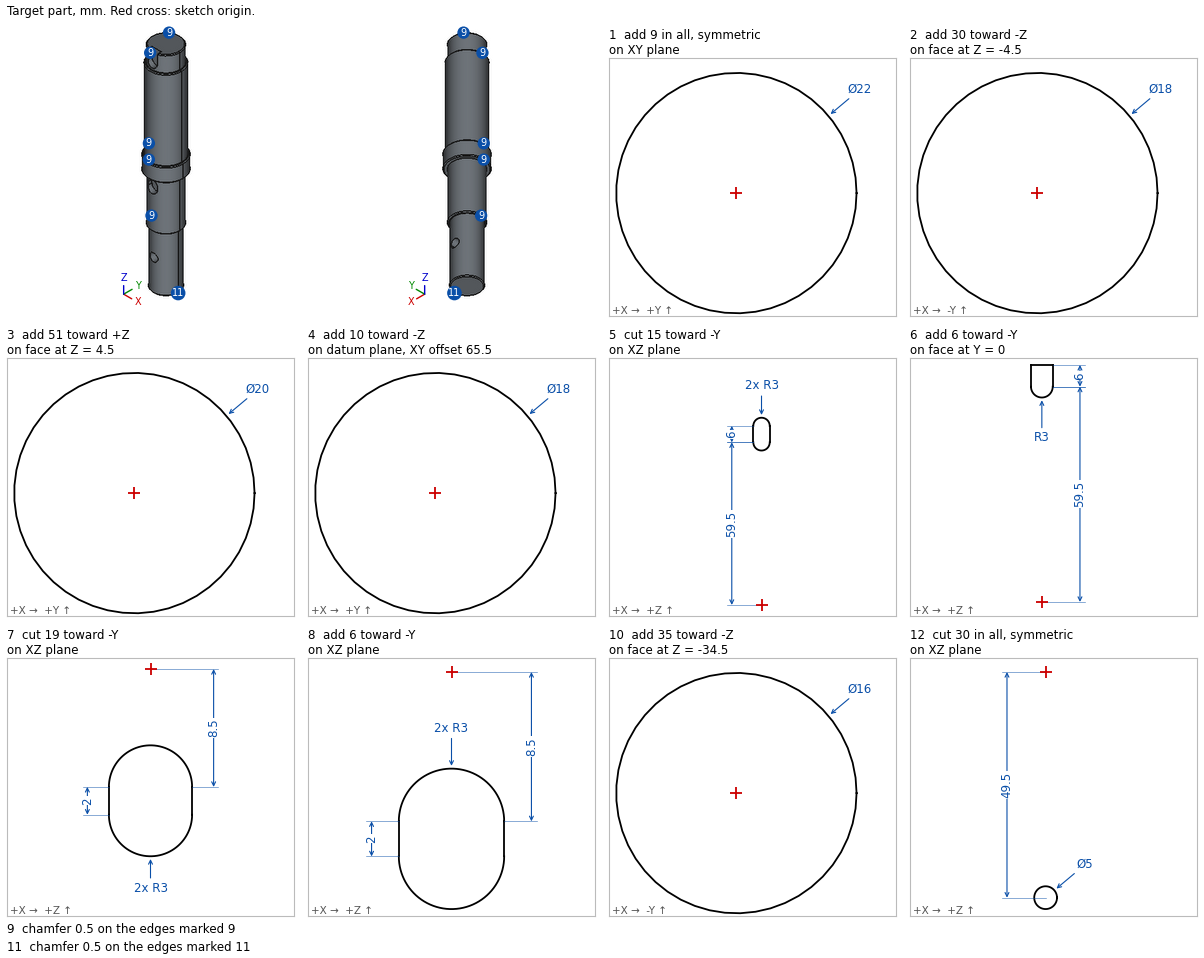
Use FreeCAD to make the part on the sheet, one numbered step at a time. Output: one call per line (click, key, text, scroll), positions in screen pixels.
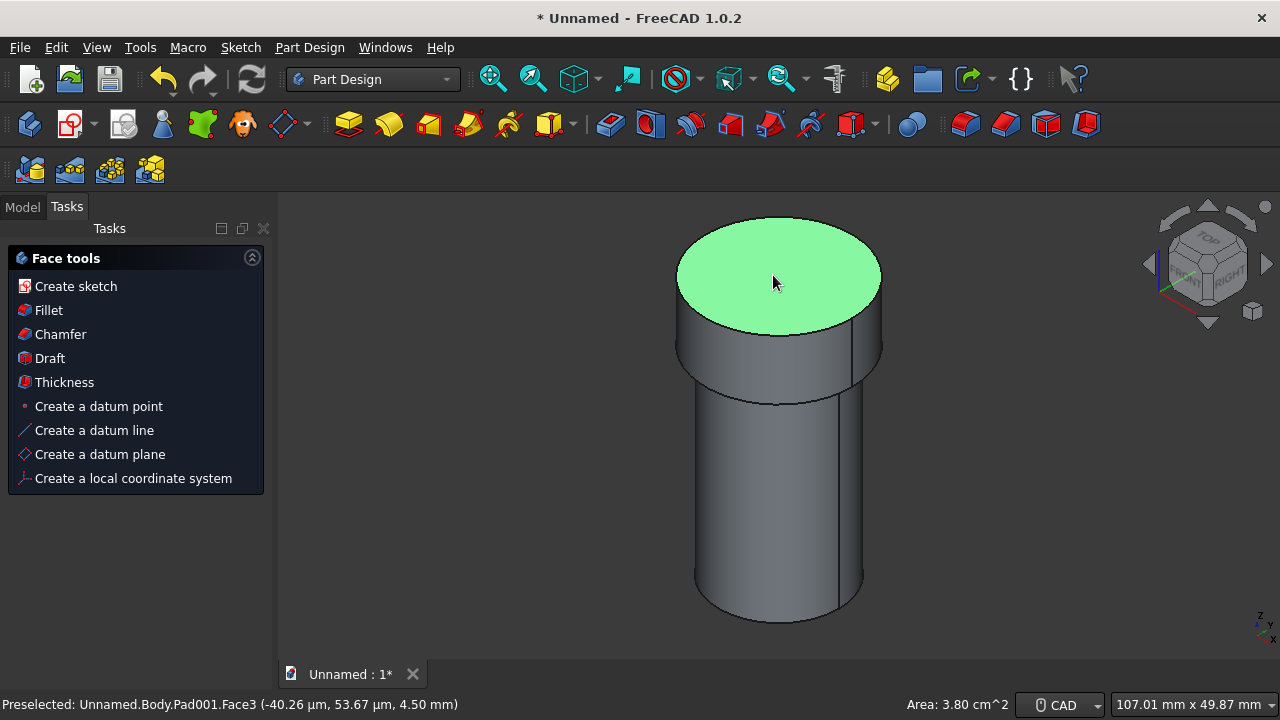
click(70, 124)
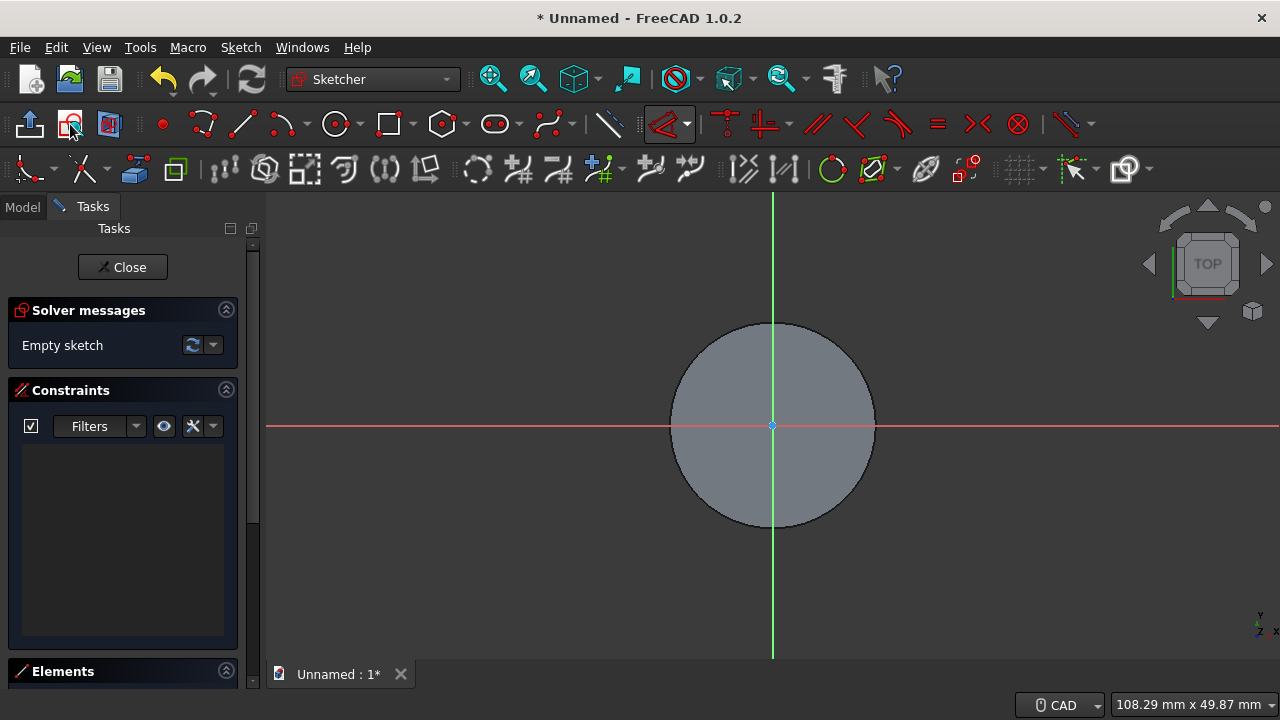
scroll(912, 425, up, 2)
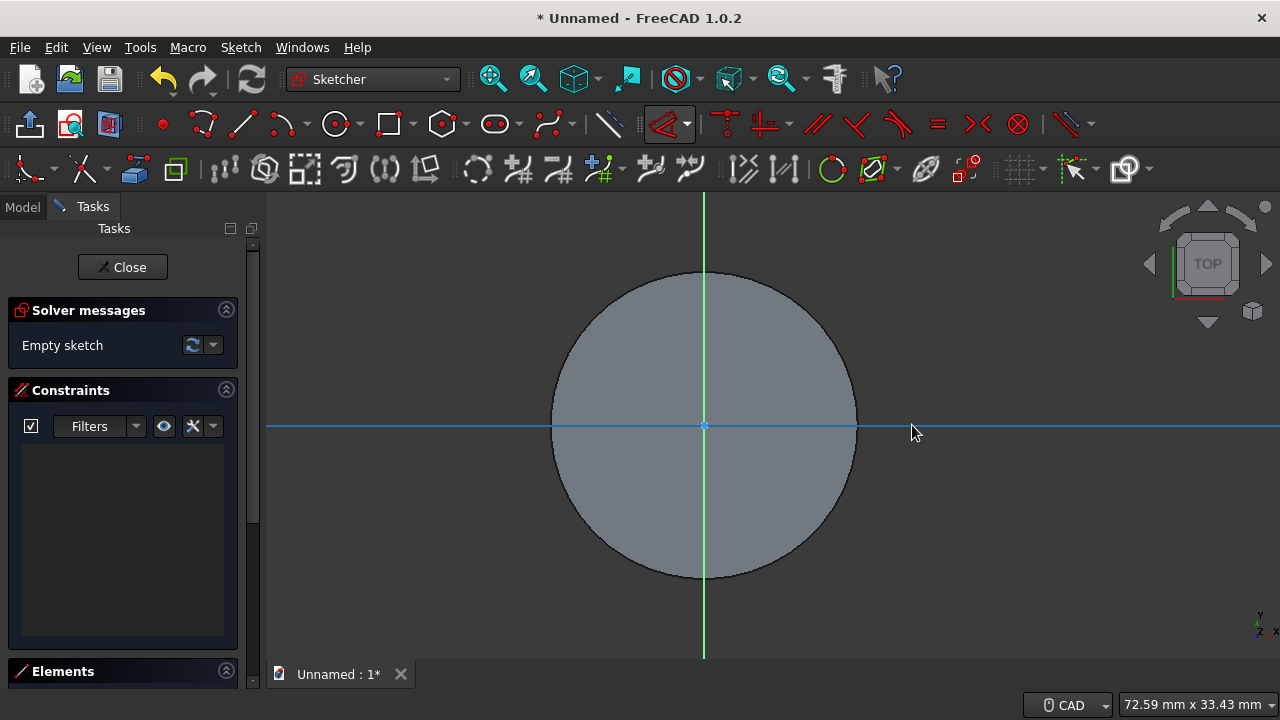
click(336, 124)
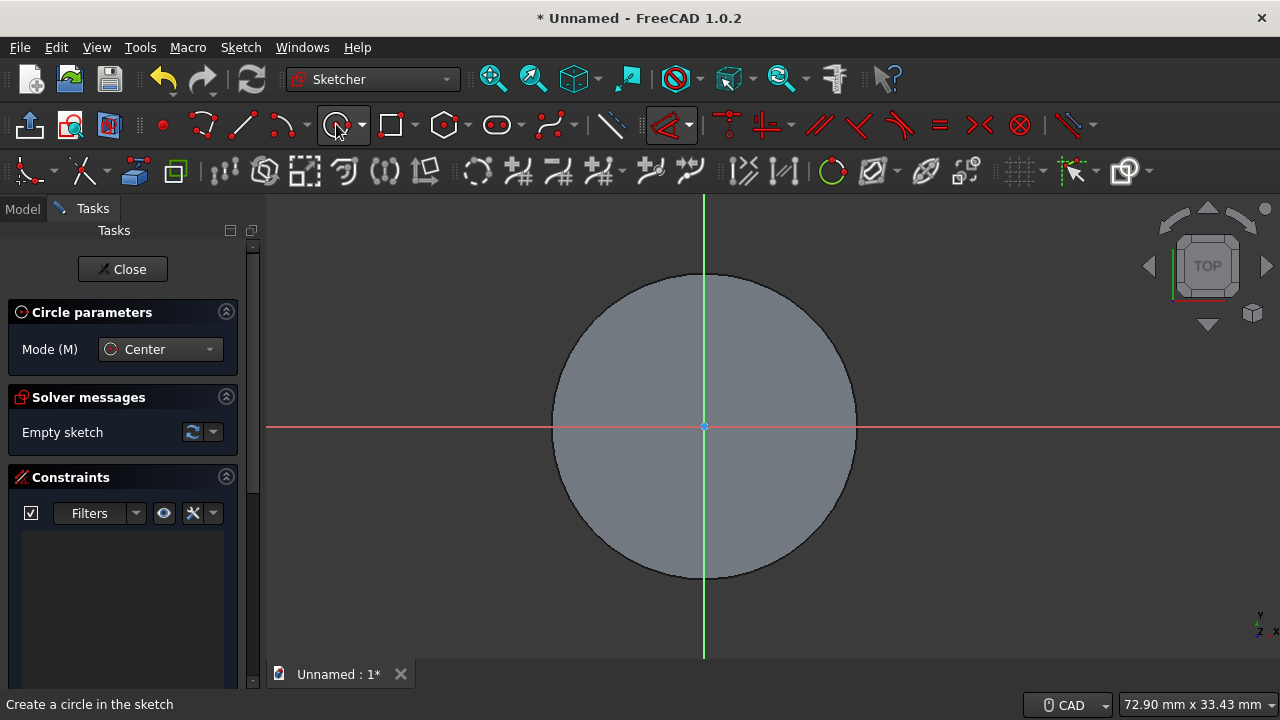
click(704, 426)
click(803, 328)
key(Escape)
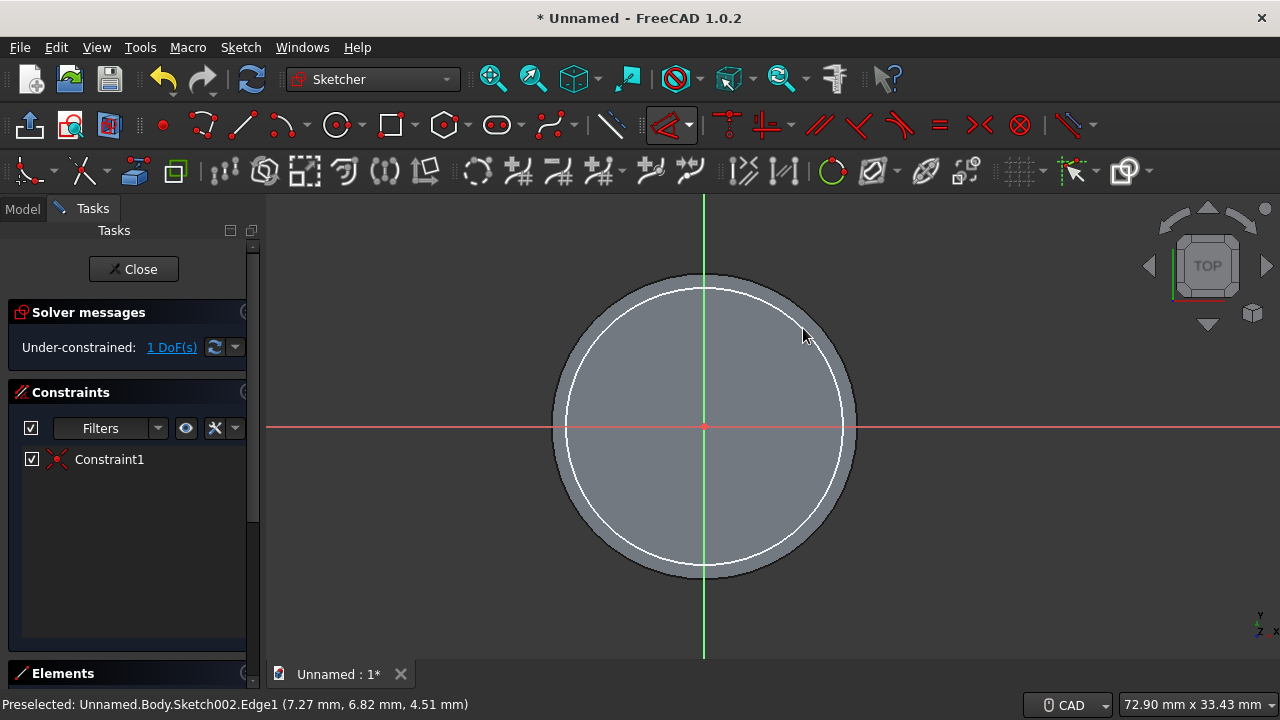
click(802, 328)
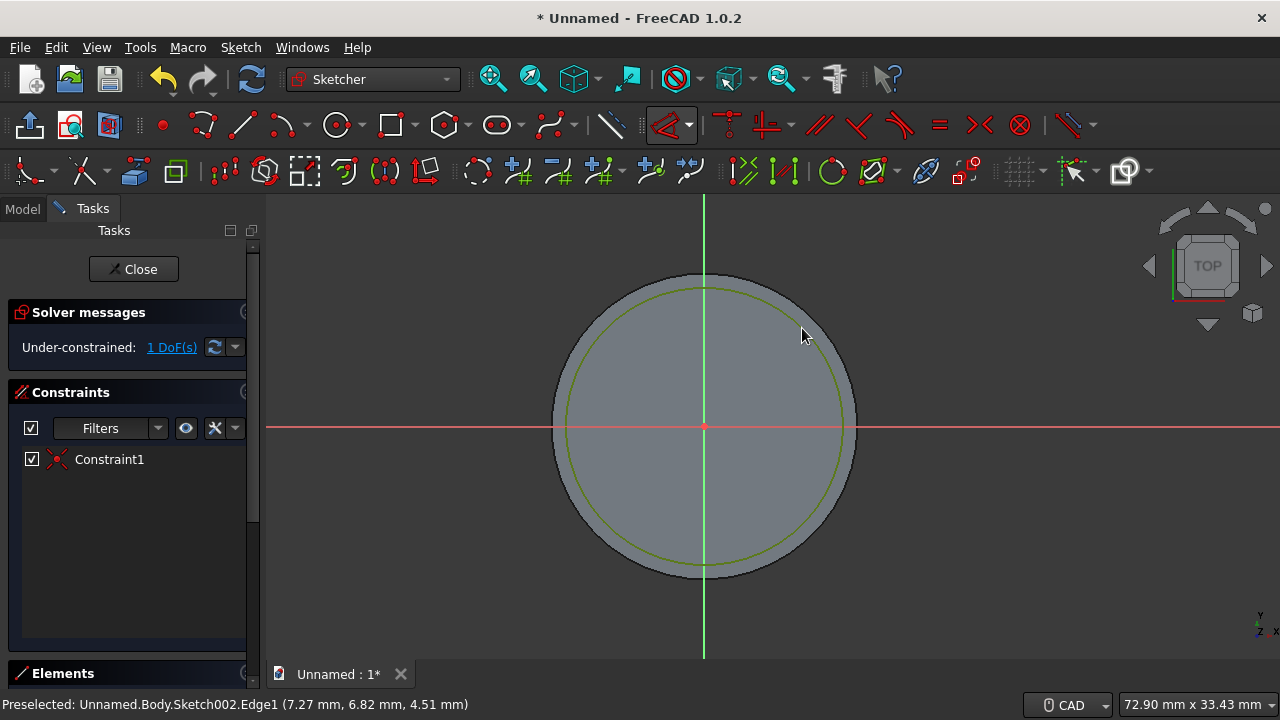
key(k)
key(o)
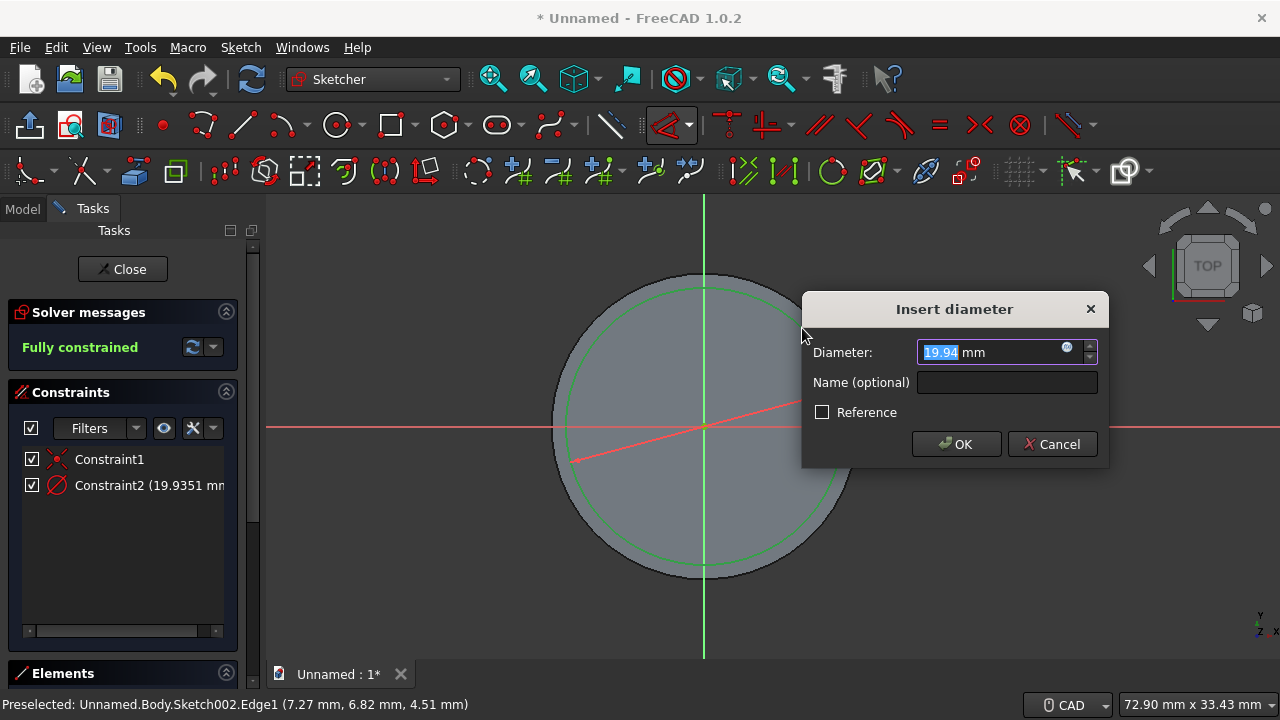
text(20)
key(Return)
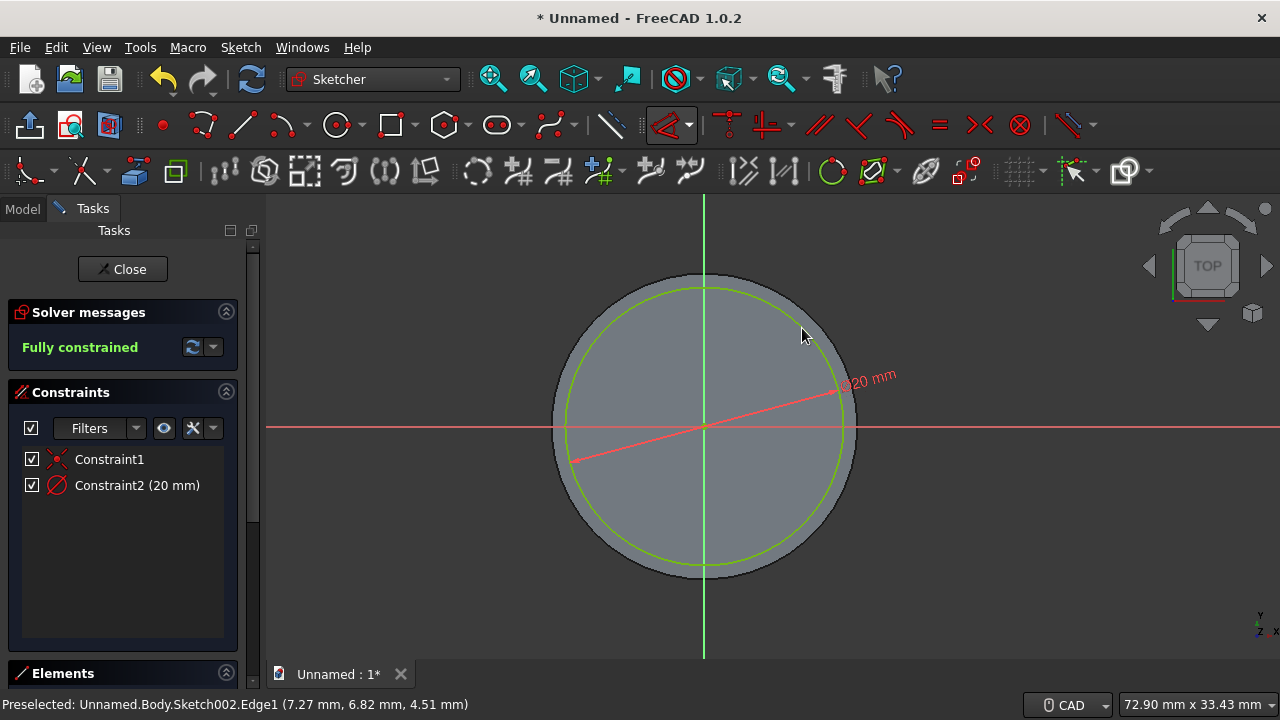
click(123, 269)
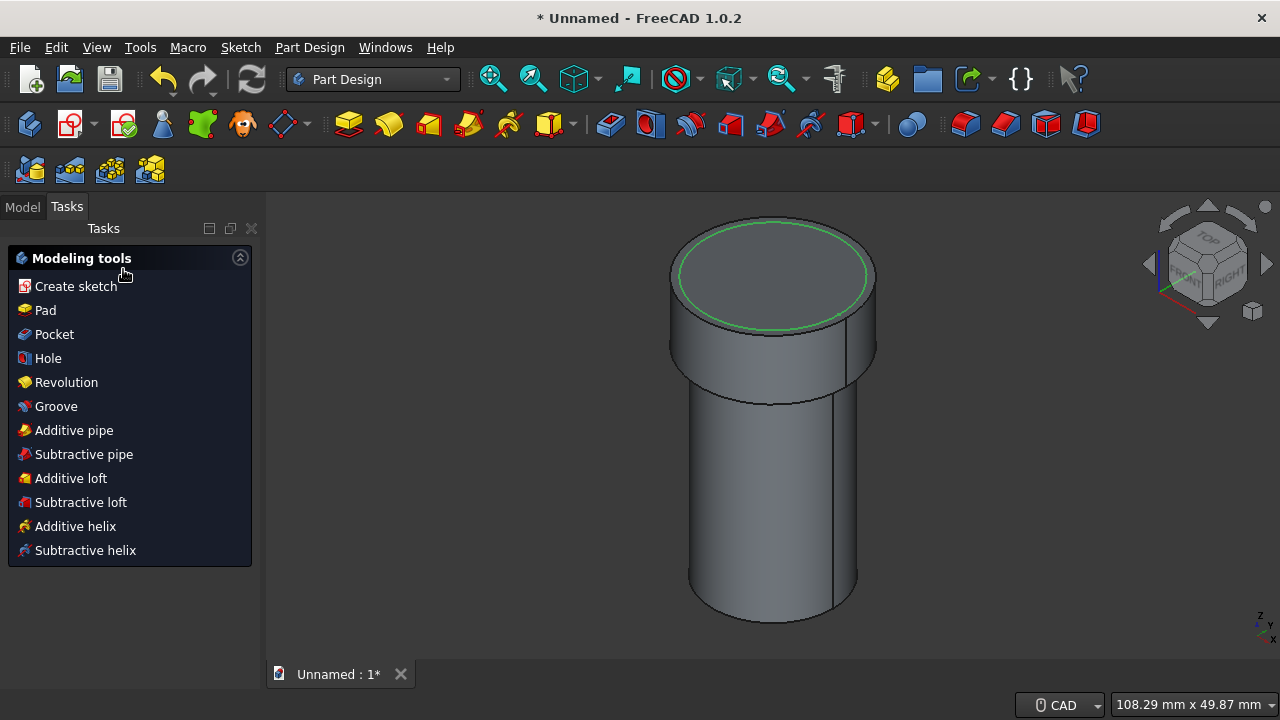
click(350, 124)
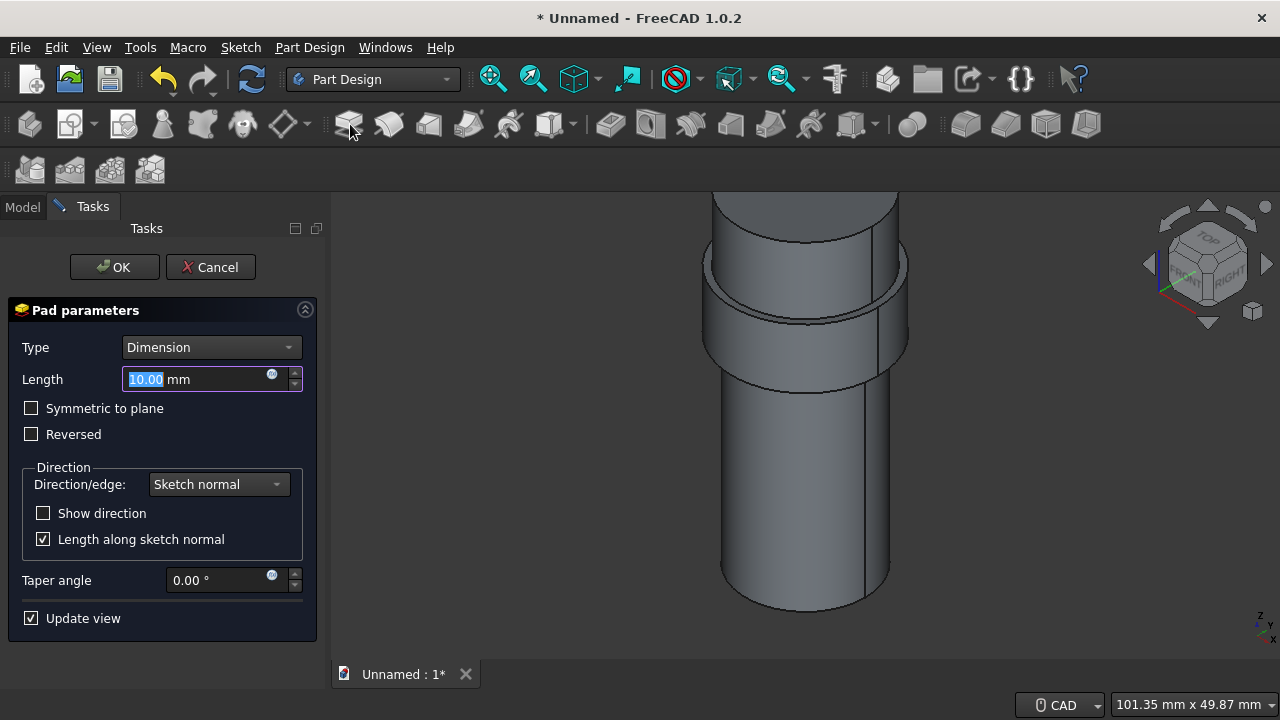
text(51)
key(Tab)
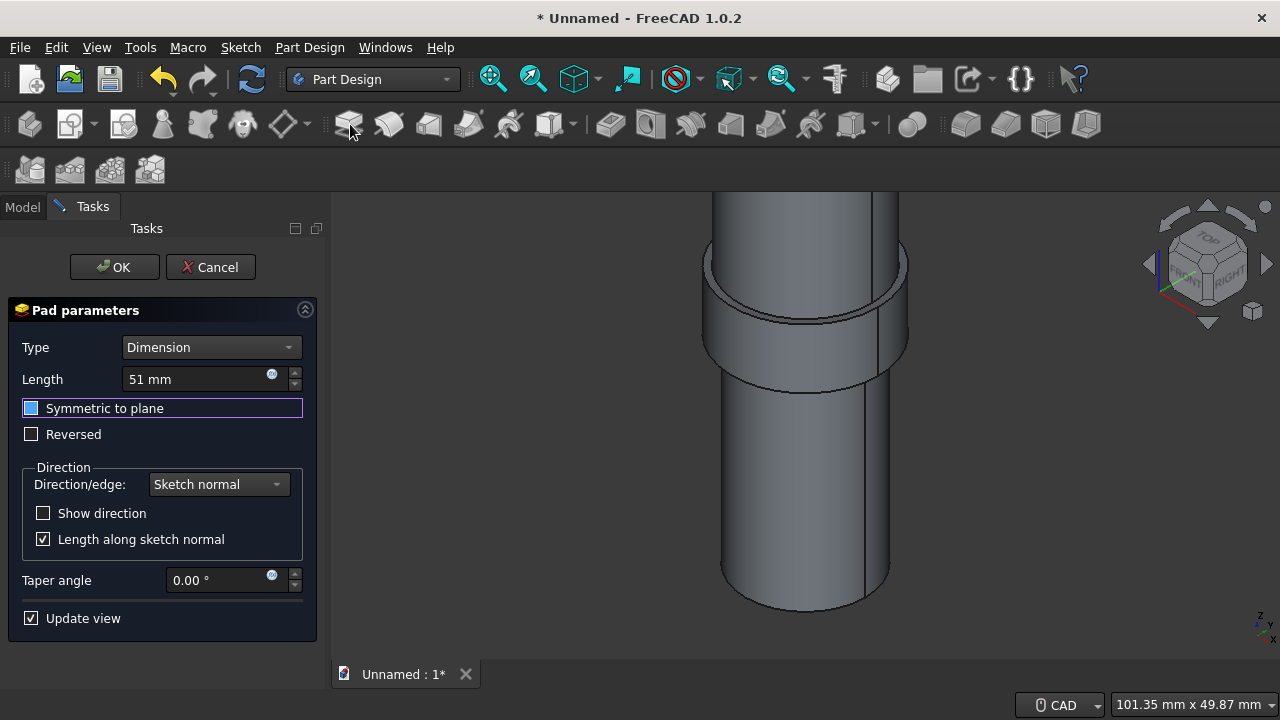
click(115, 267)